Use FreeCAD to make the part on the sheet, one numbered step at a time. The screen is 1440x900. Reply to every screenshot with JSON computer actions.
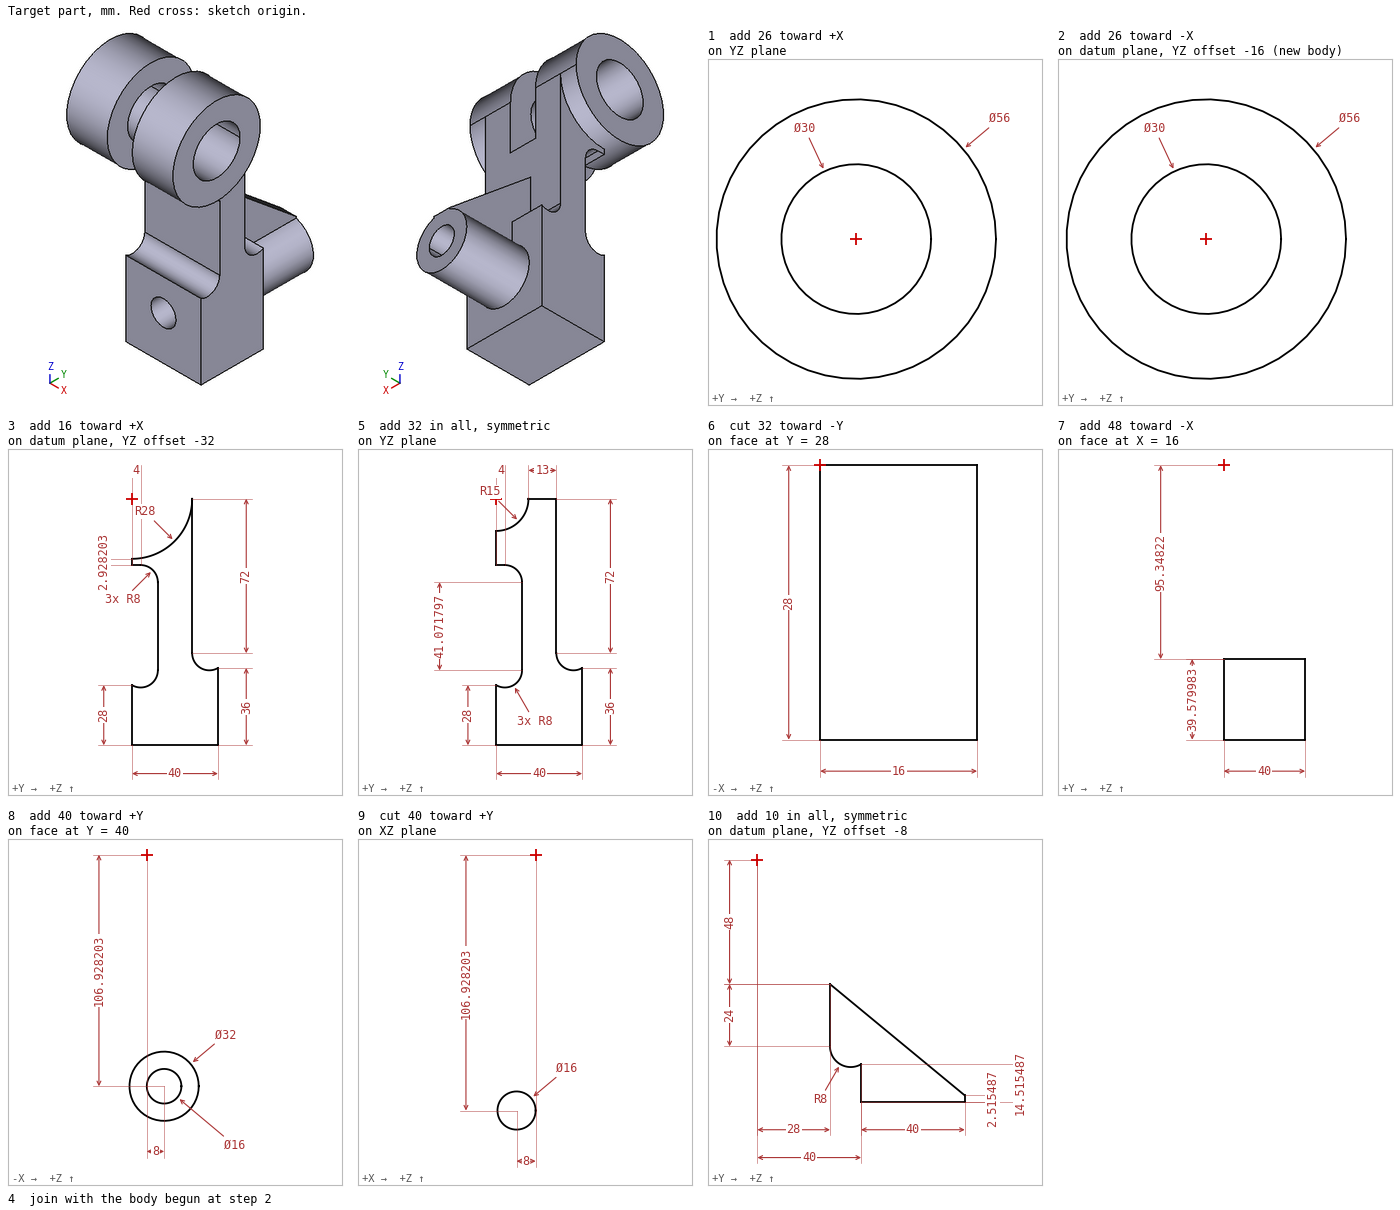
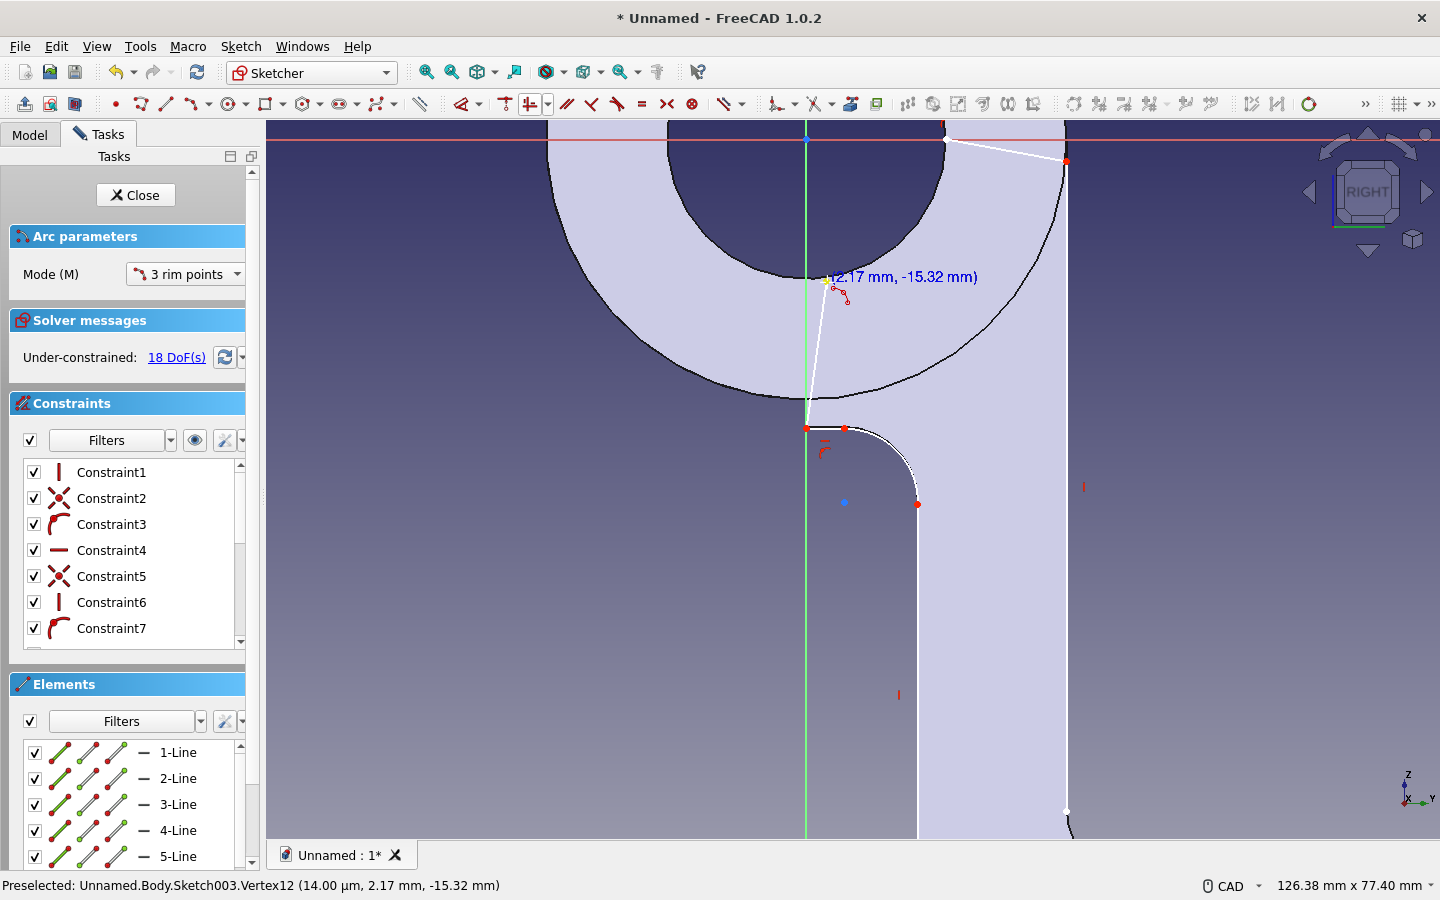
{"action": "scroll", "coordinate": [615, 321], "scroll_direction": "down", "scroll_amount": 4}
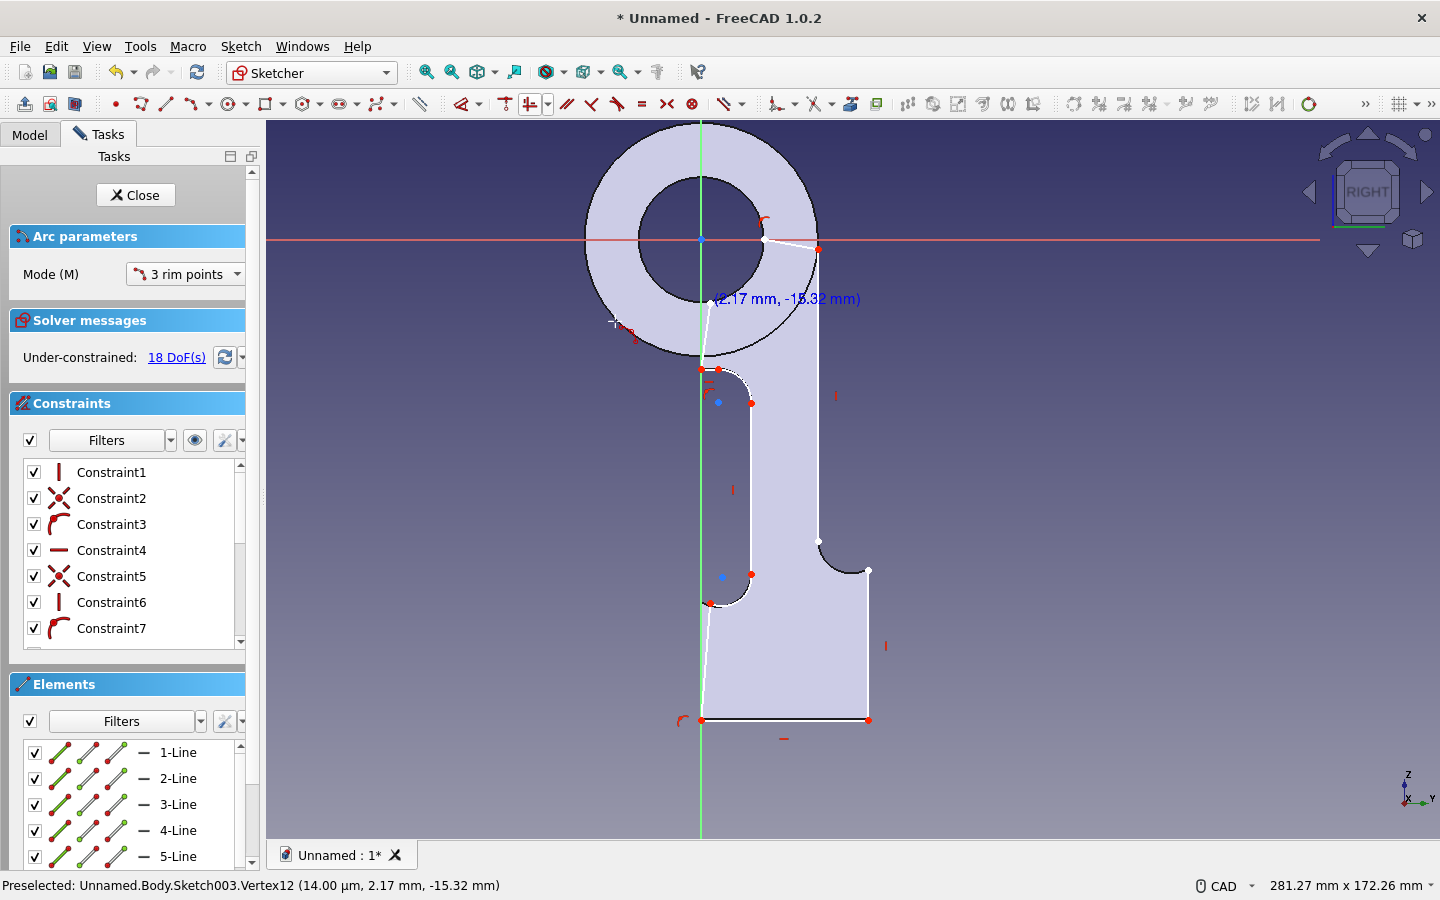
{"action": "left_click", "coordinate": [764, 240]}
{"action": "left_click", "coordinate": [745, 284]}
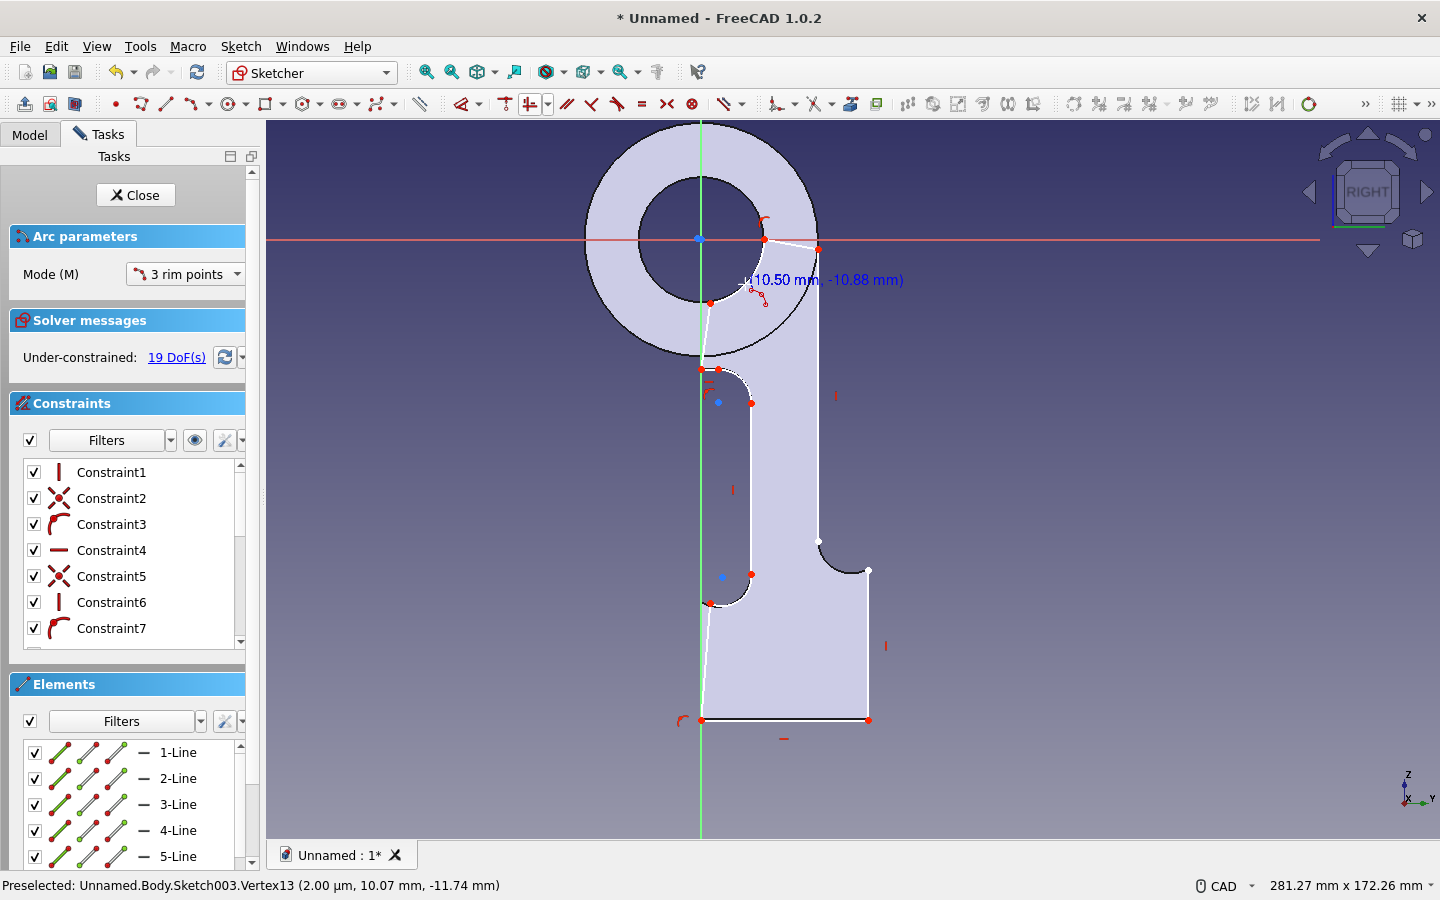
{"action": "left_click", "coordinate": [818, 542]}
{"action": "left_click", "coordinate": [868, 571]}
{"action": "left_click", "coordinate": [835, 569]}
{"action": "key", "text": "Escape"}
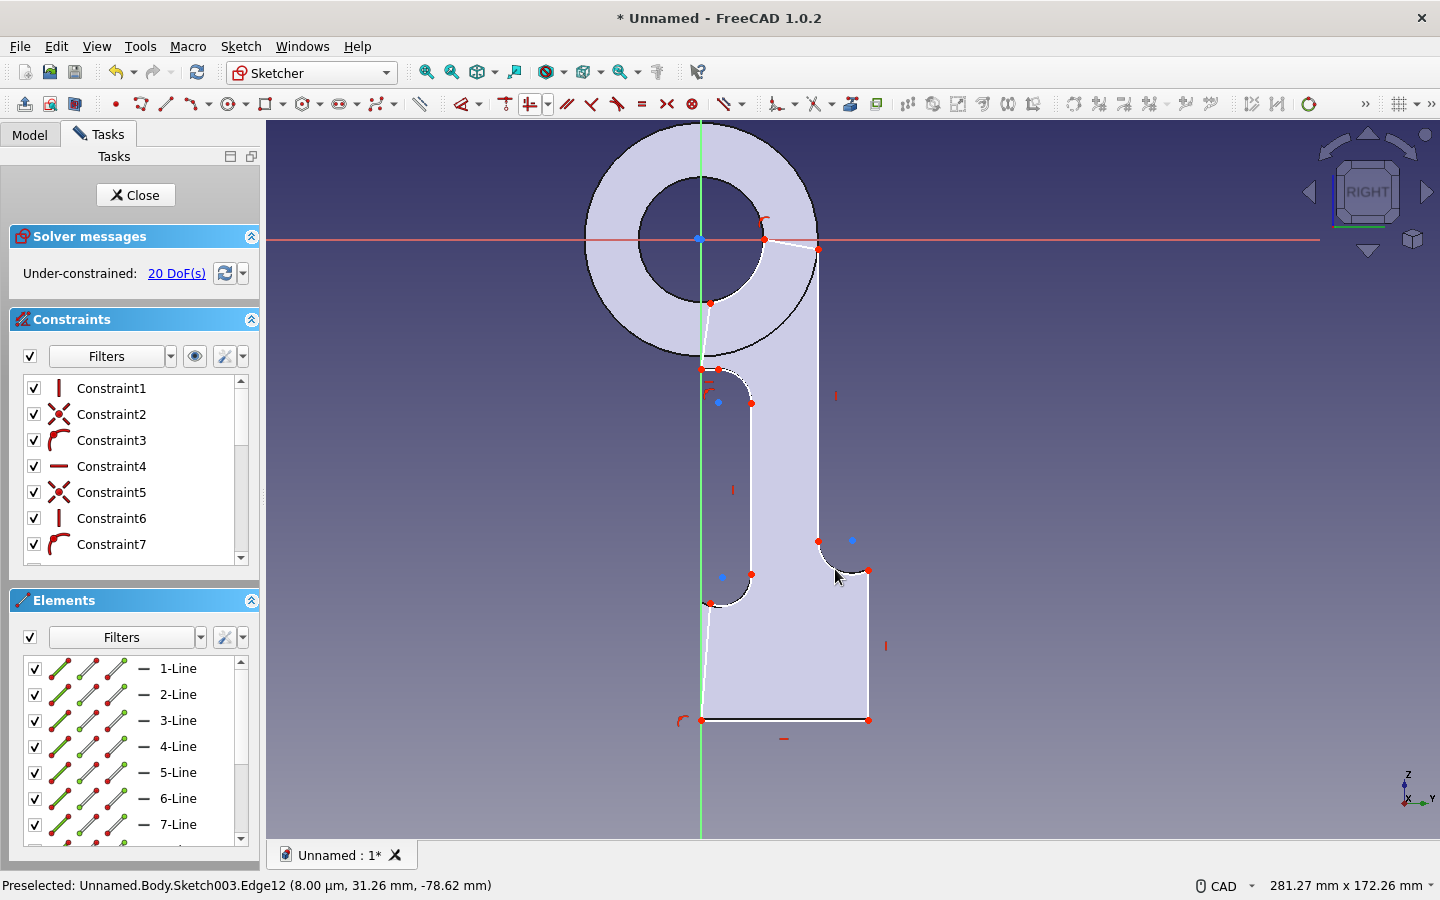
{"action": "left_click", "coordinate": [751, 523]}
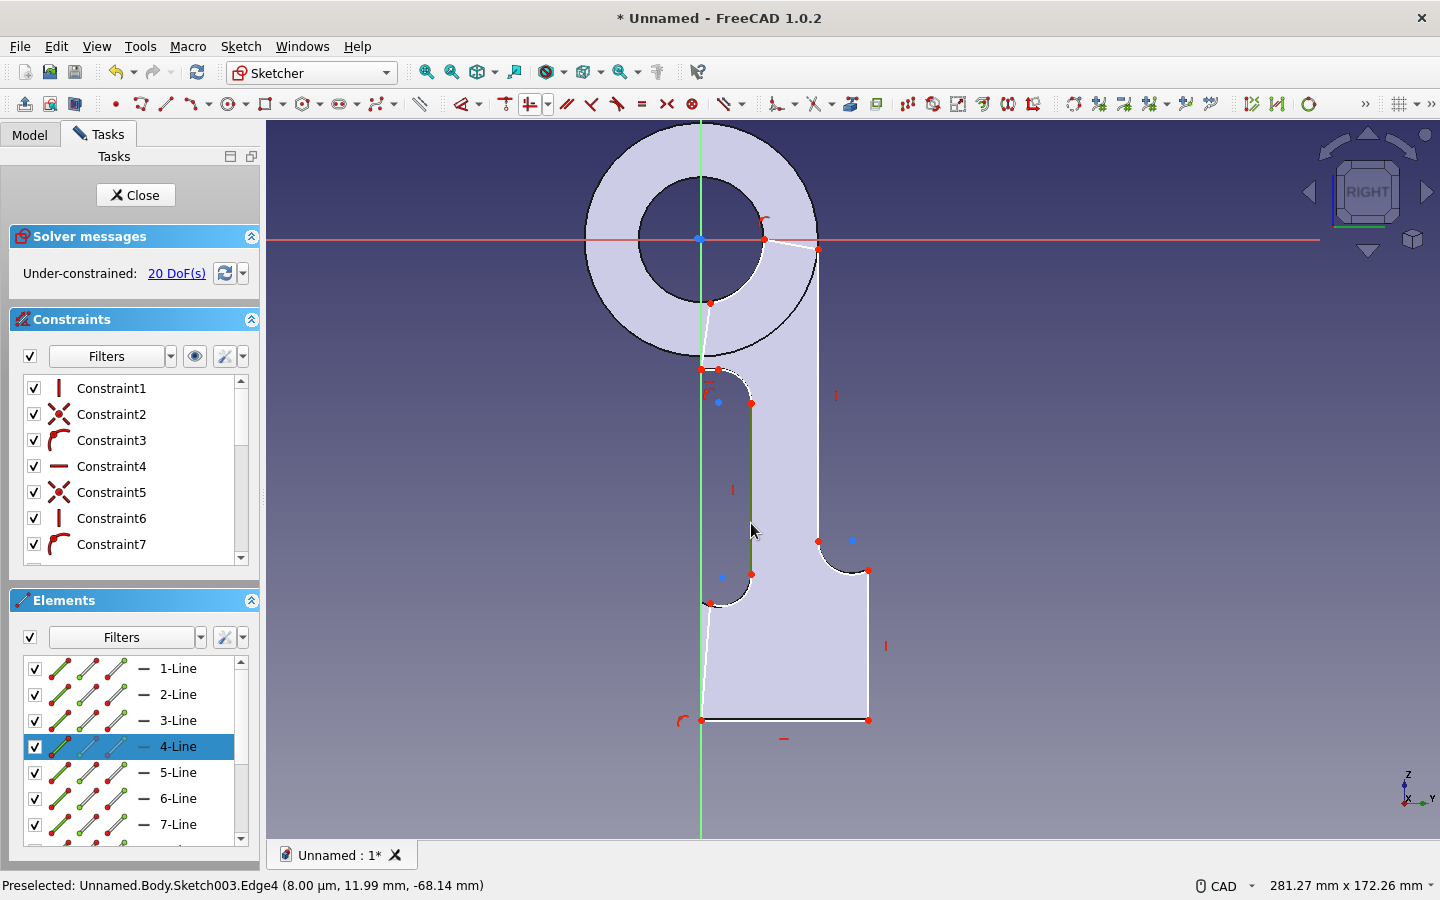
{"action": "left_click", "coordinate": [728, 606]}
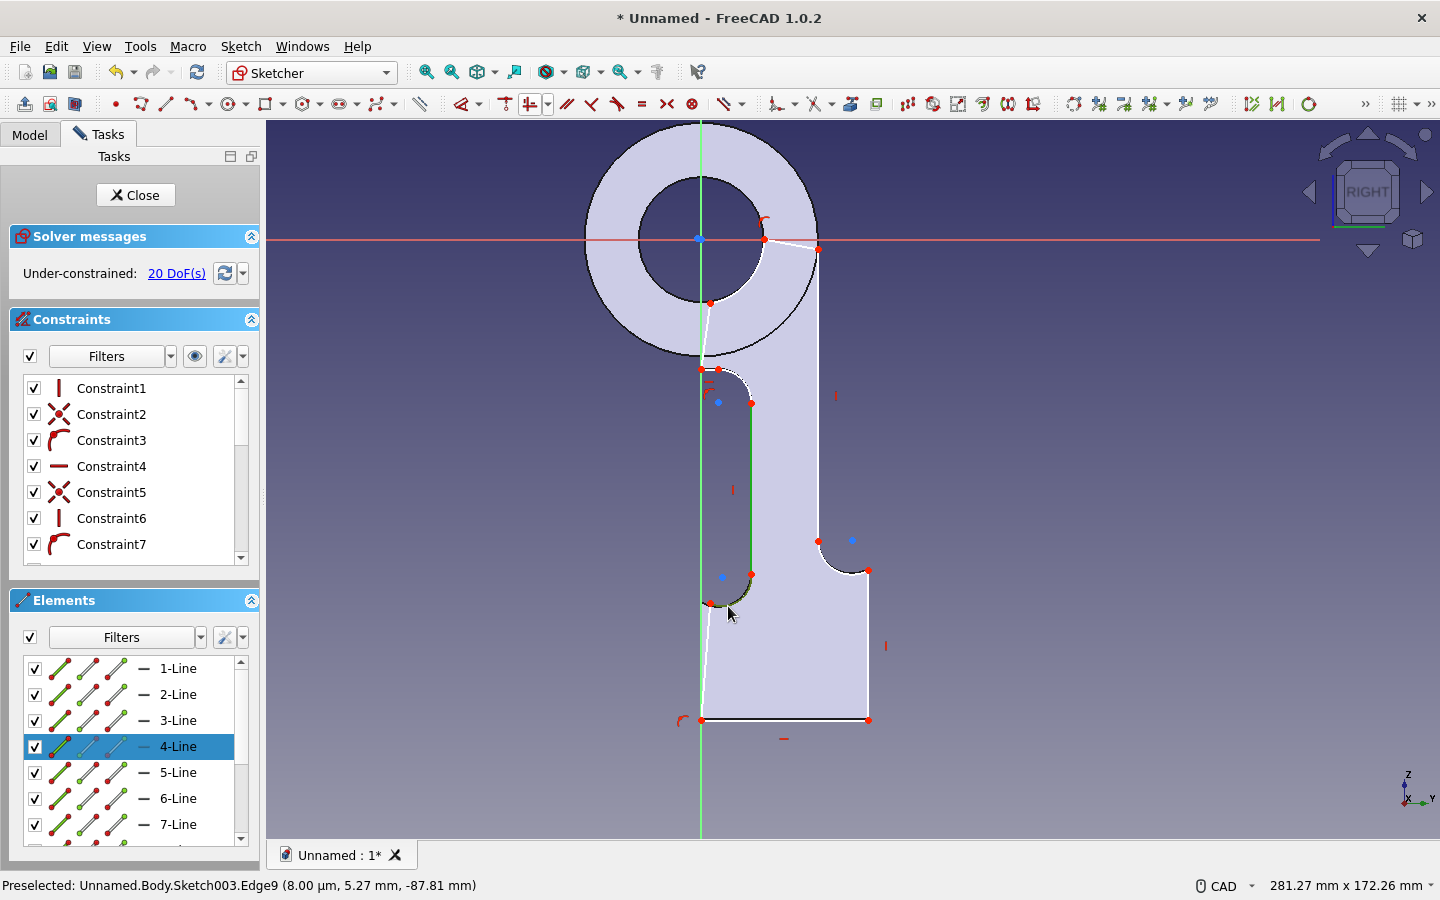
{"action": "left_click", "coordinate": [617, 104]}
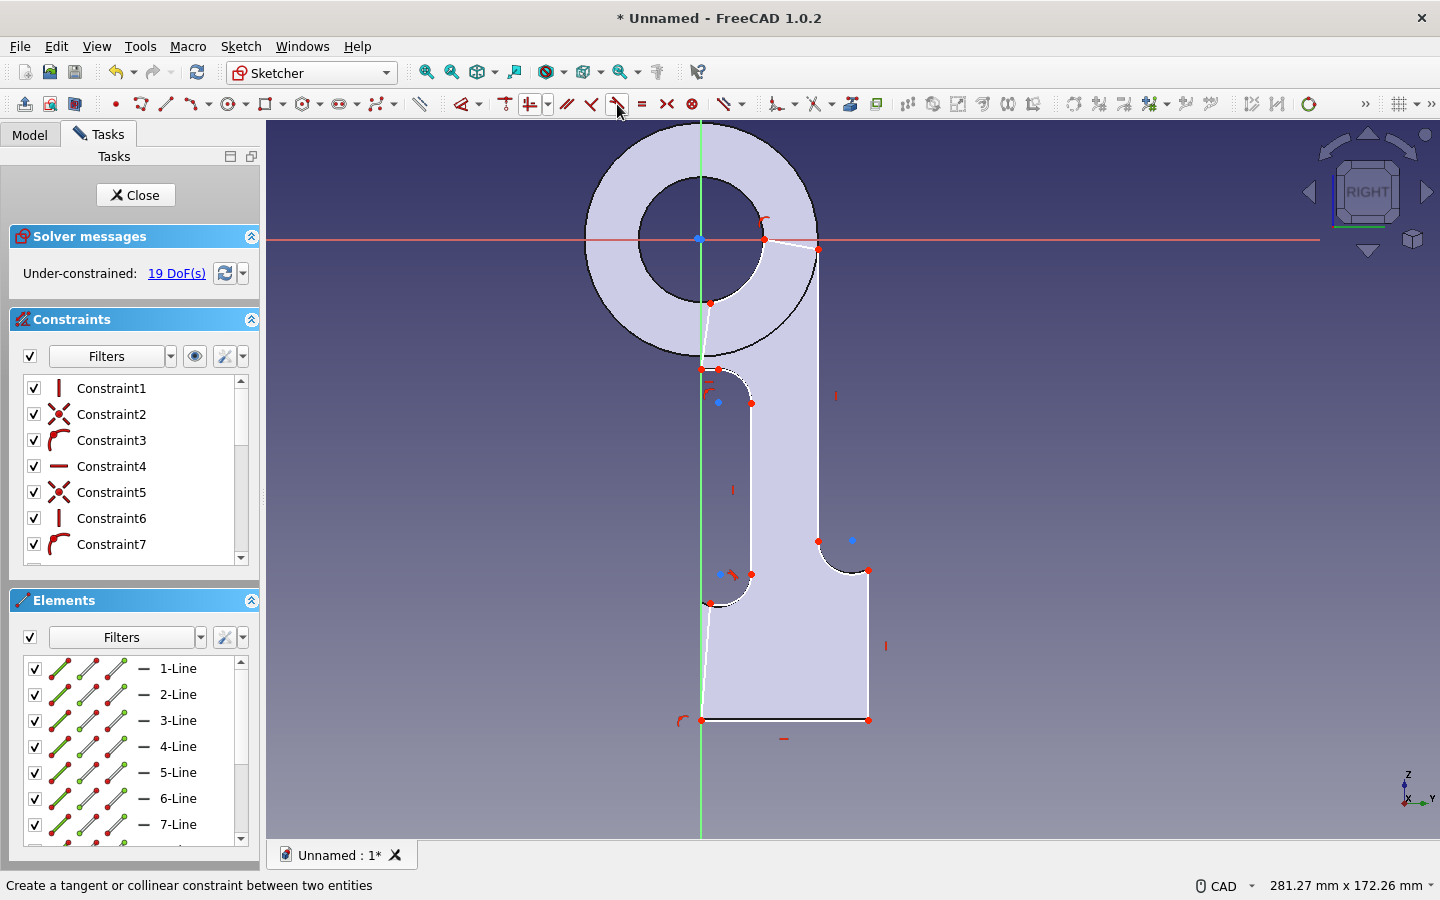
{"action": "left_click", "coordinate": [751, 523]}